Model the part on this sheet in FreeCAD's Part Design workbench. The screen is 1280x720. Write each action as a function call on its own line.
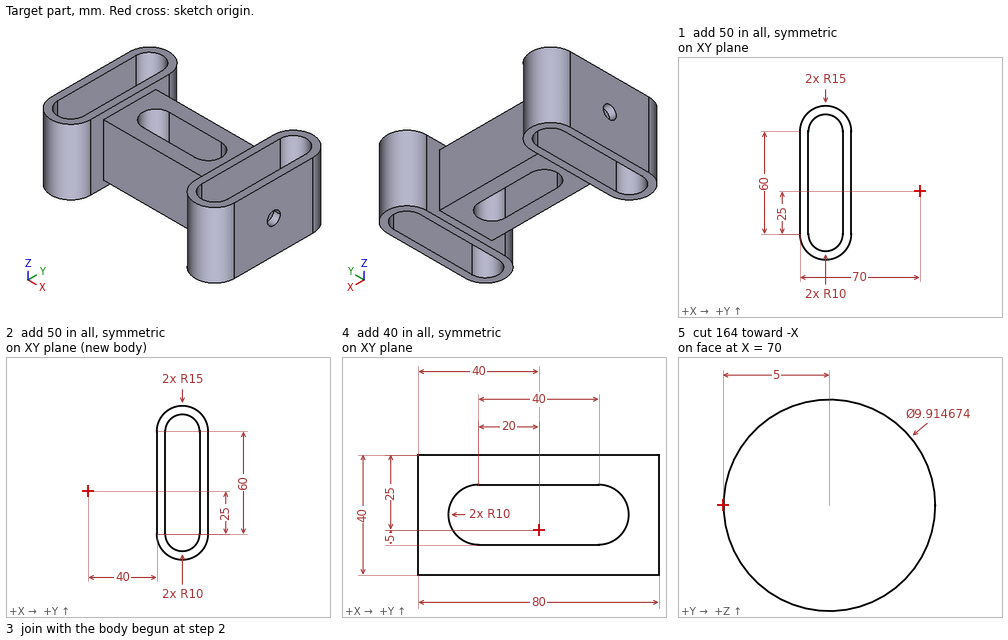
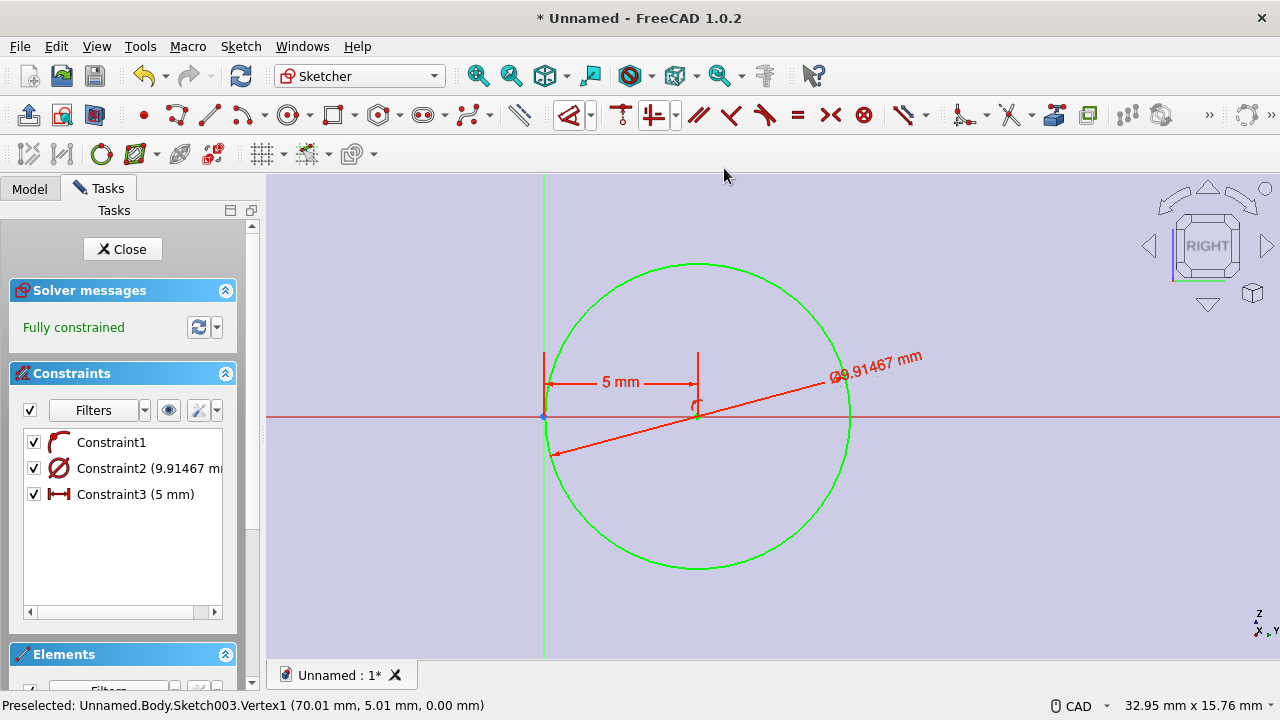
click(123, 249)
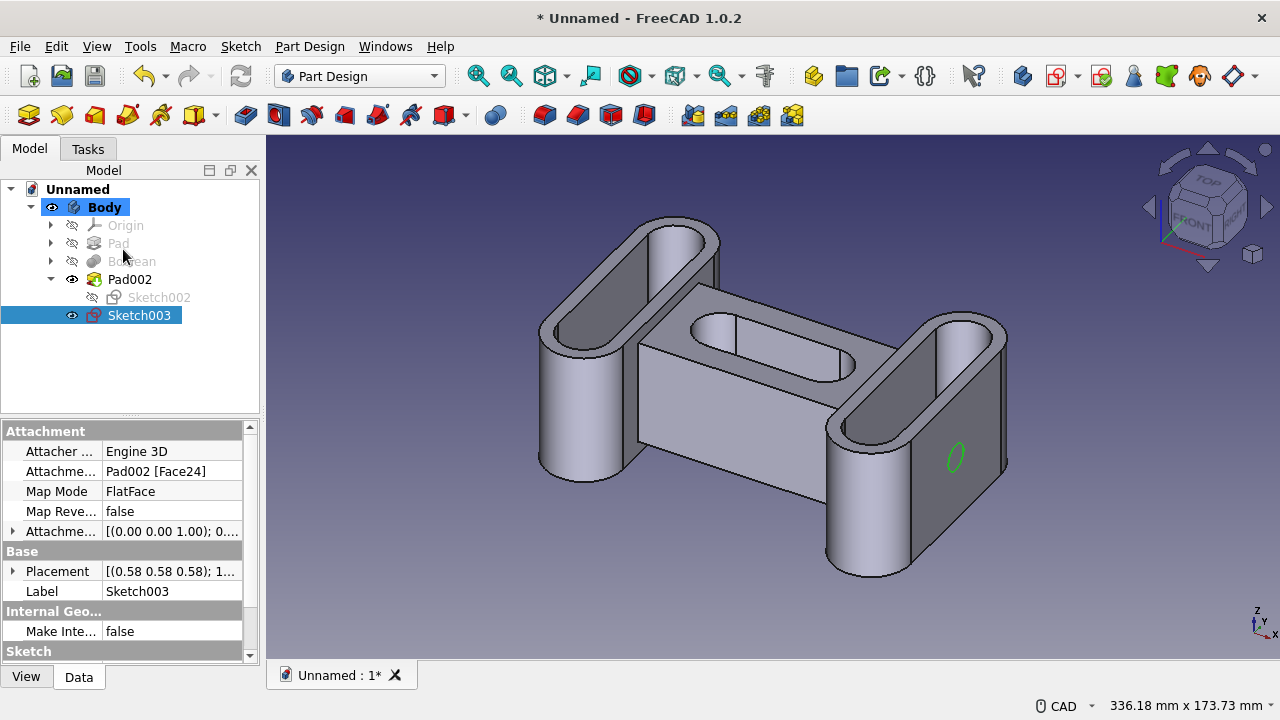
click(246, 116)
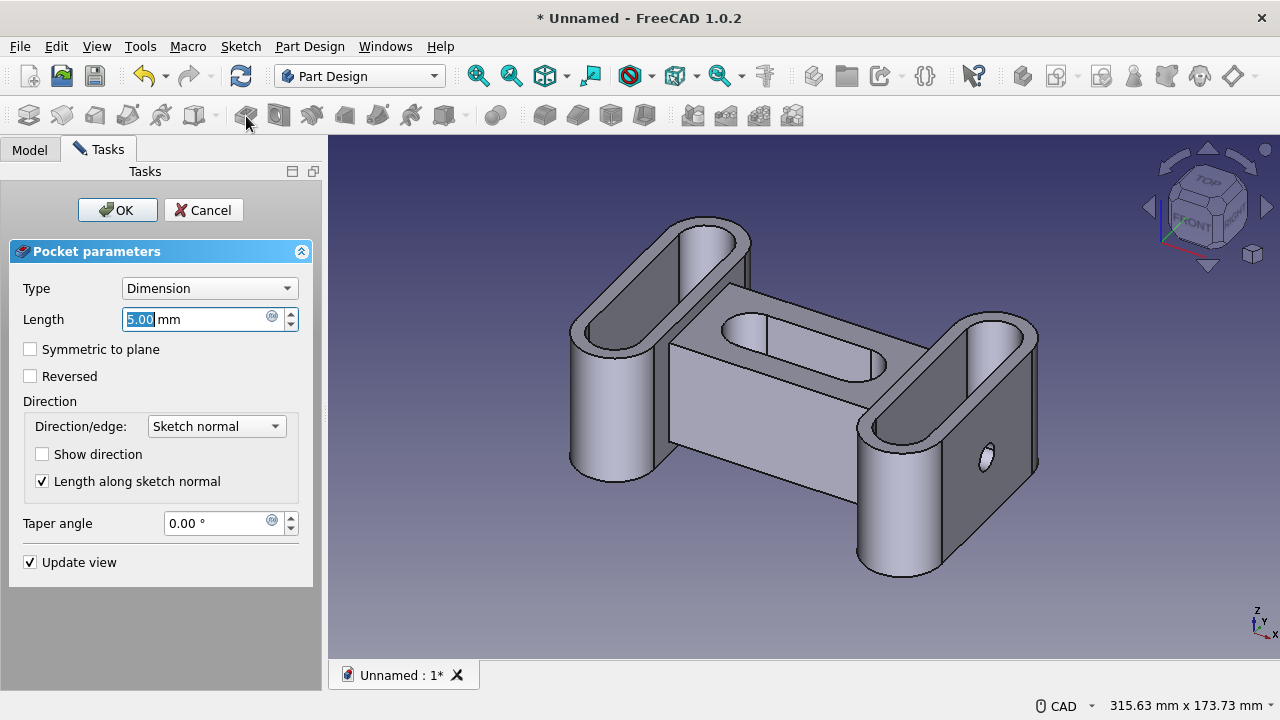
text(164)
key(Tab)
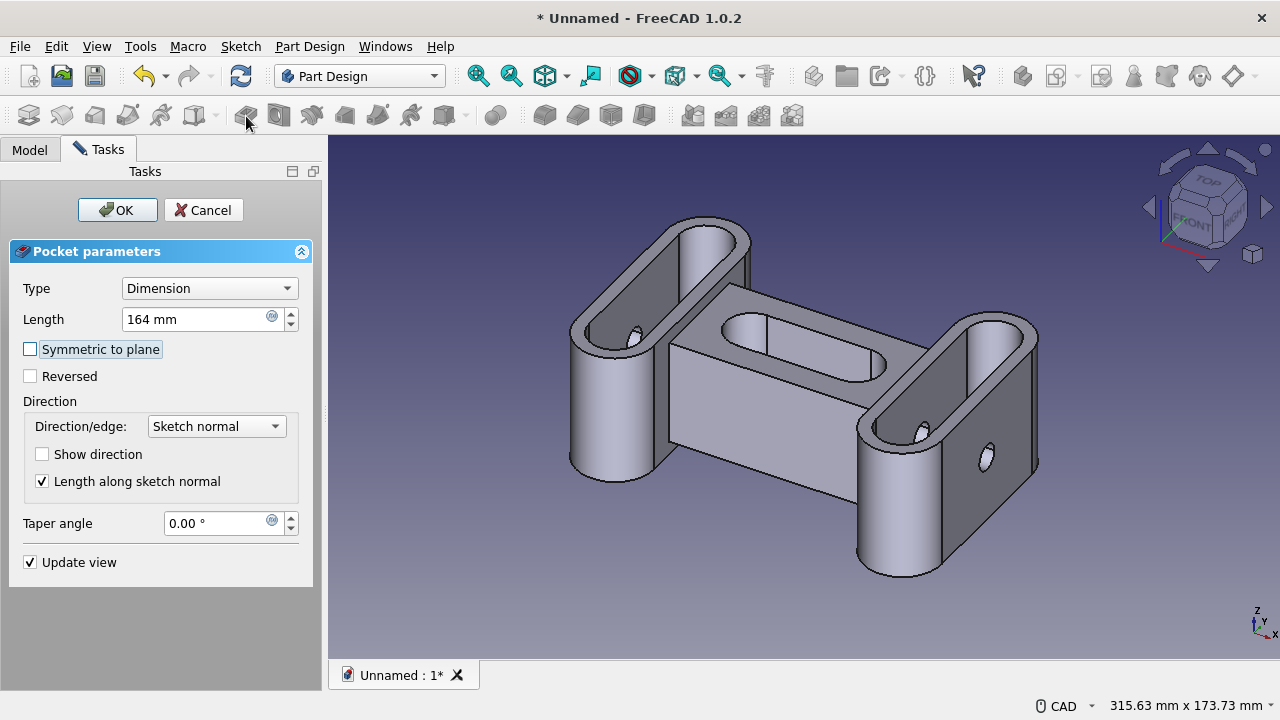
click(118, 210)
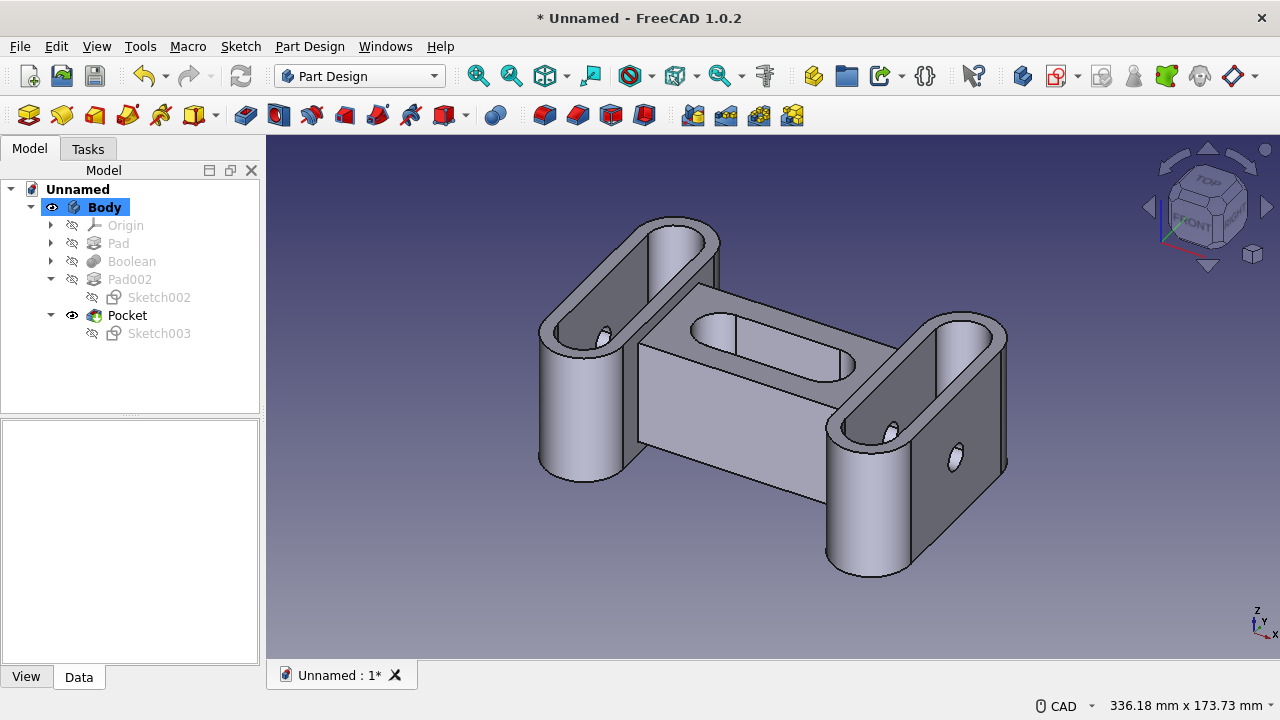
key(0)